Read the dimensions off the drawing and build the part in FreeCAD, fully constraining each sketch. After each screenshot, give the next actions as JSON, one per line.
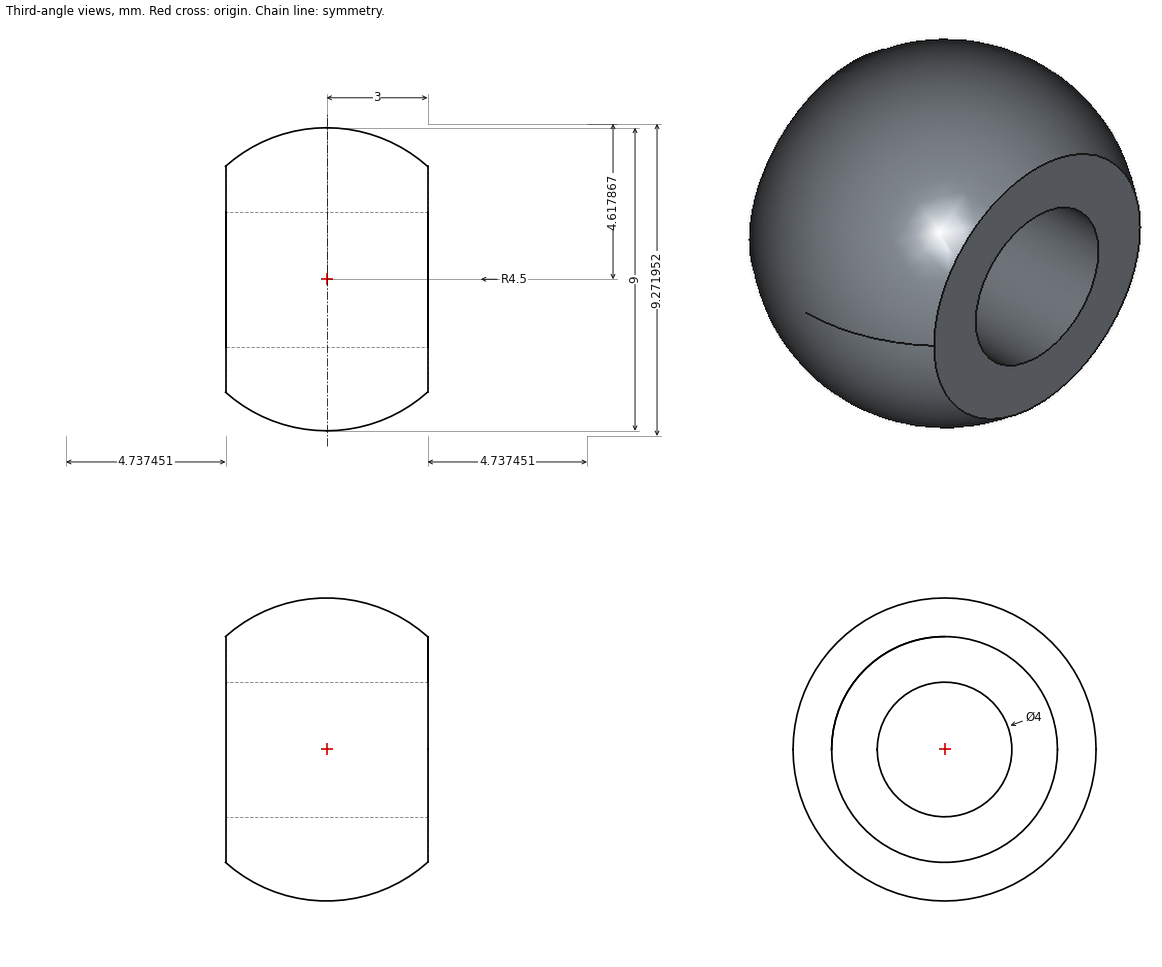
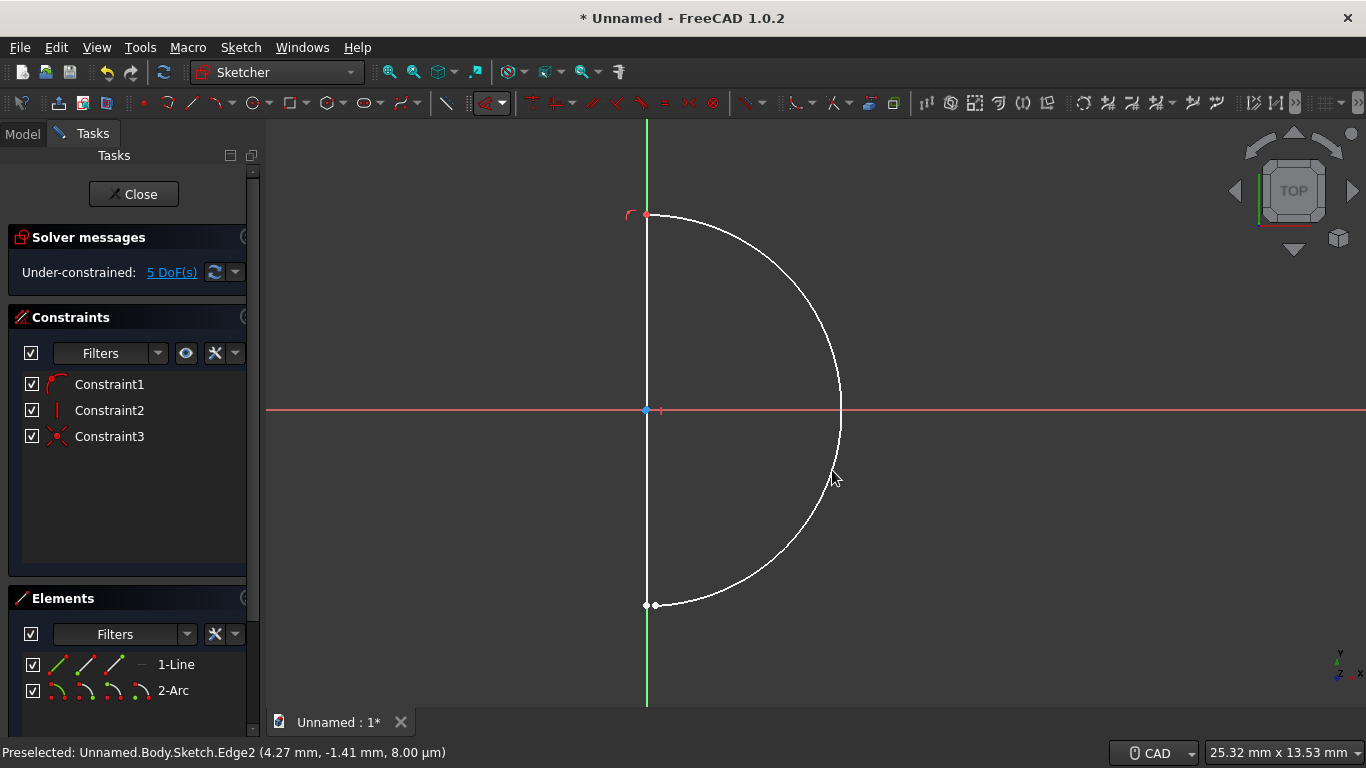
{"action": "left_click_drag", "start_coordinate": [636, 400], "coordinate": [657, 421]}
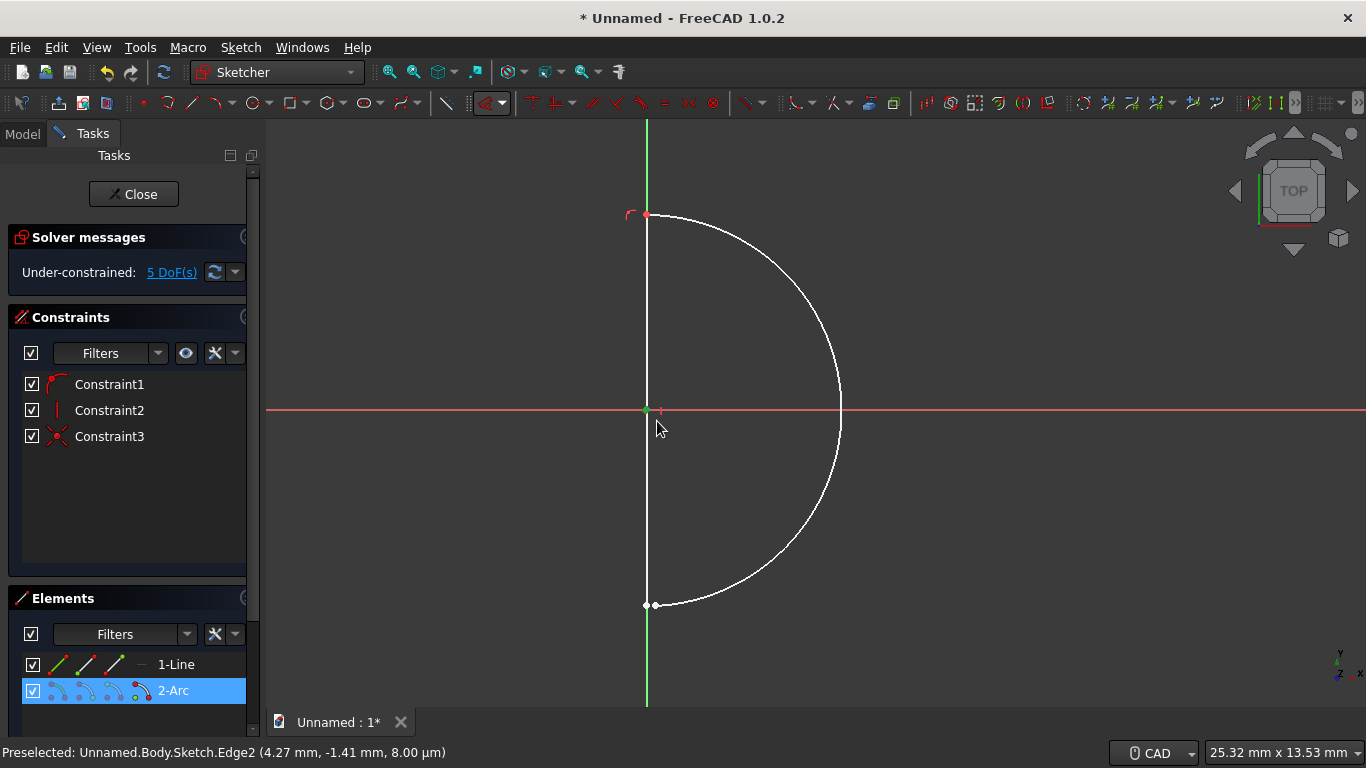
{"action": "key", "text": "c"}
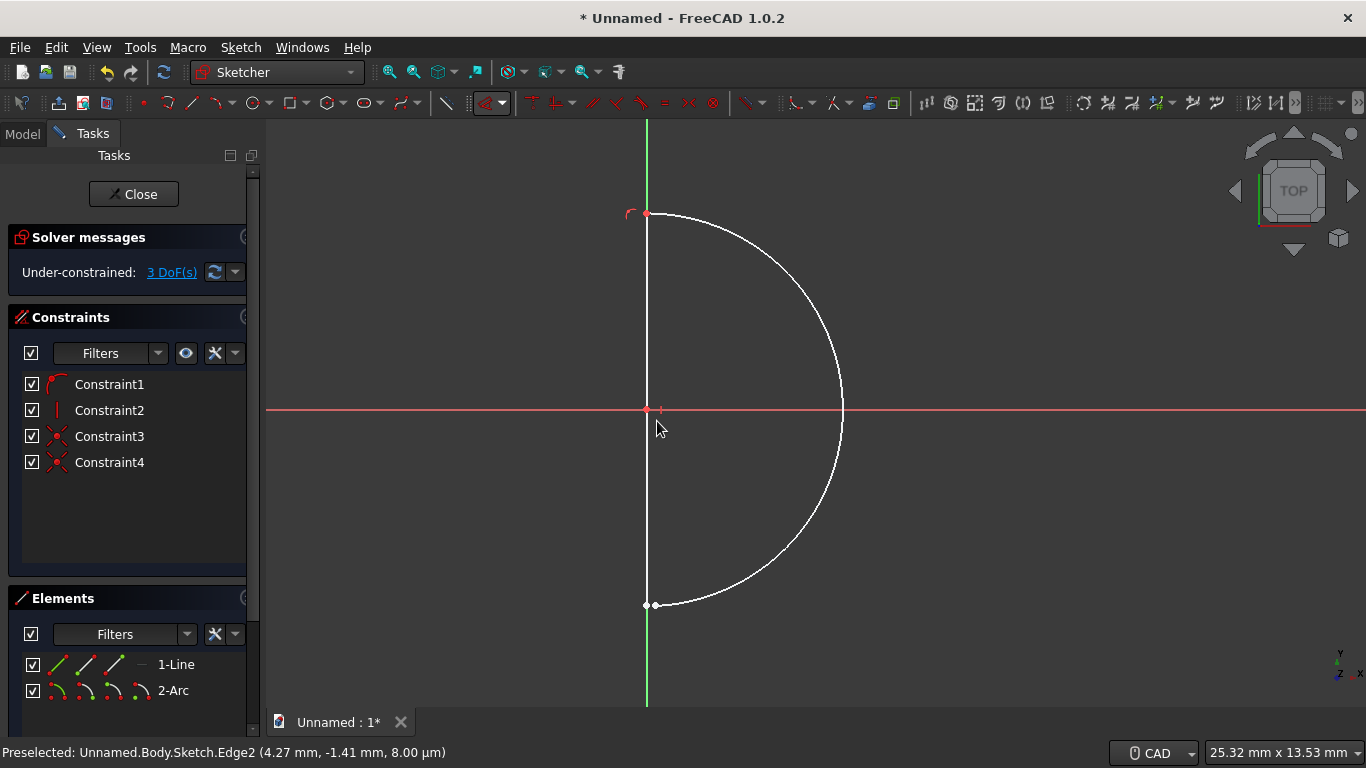
{"action": "left_click", "coordinate": [486, 104]}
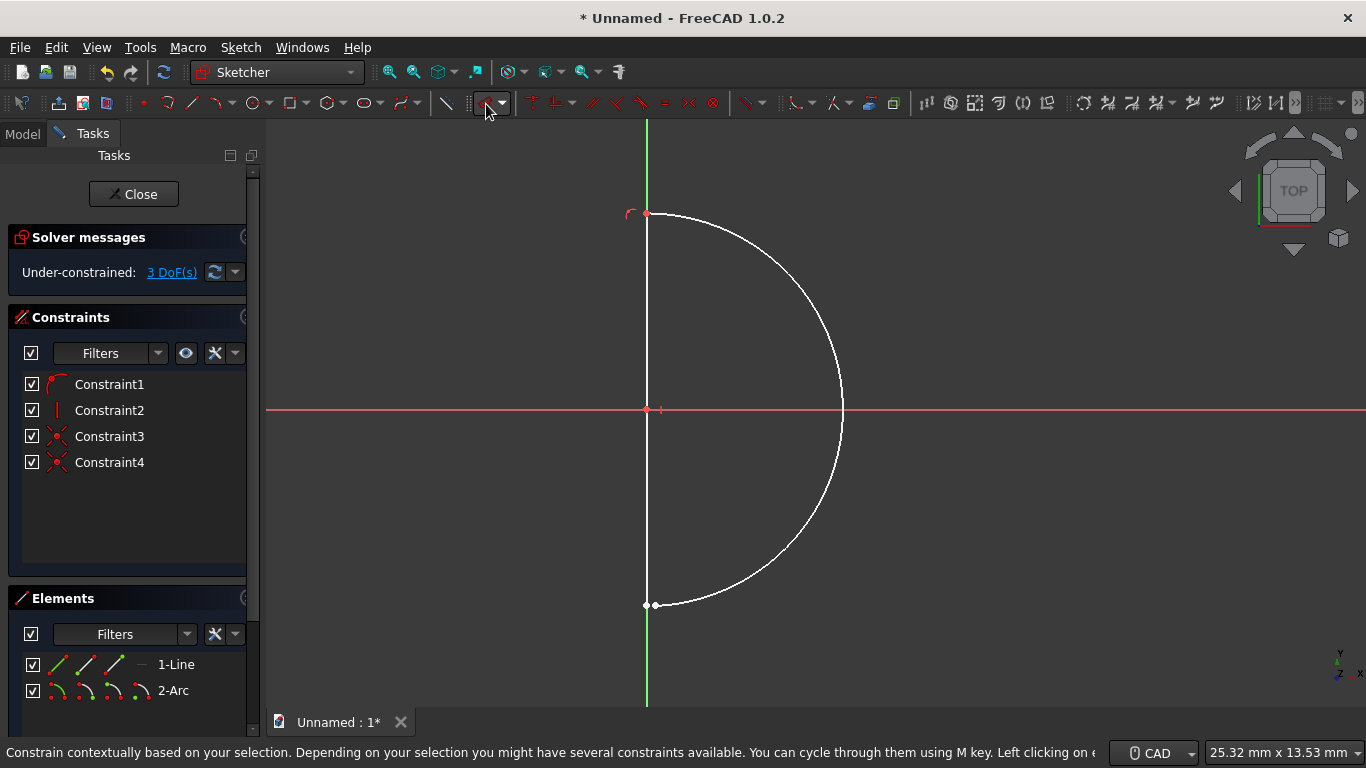
{"action": "left_click", "coordinate": [809, 520]}
{"action": "left_click", "coordinate": [835, 538]}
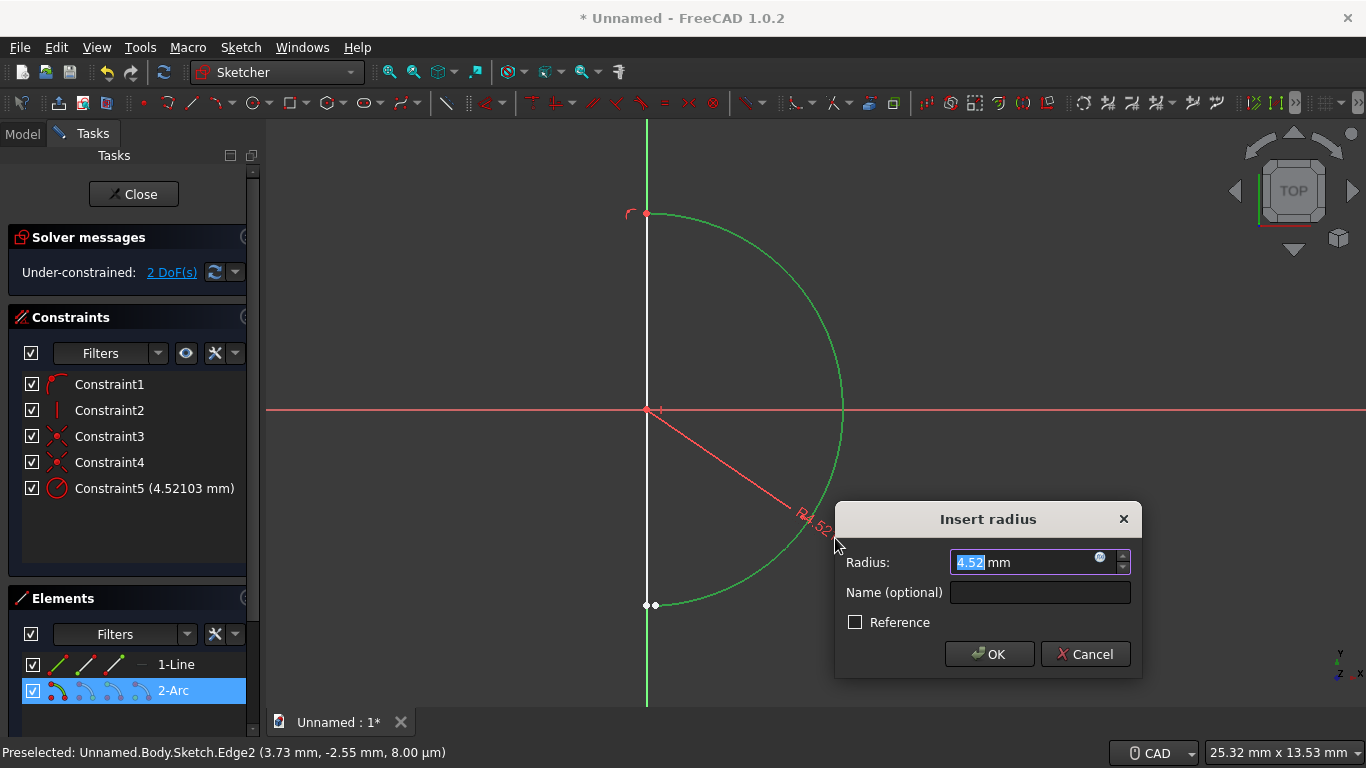
{"action": "type", "text": "4.5"}
{"action": "key", "text": "Return"}
{"action": "key", "text": "Escape"}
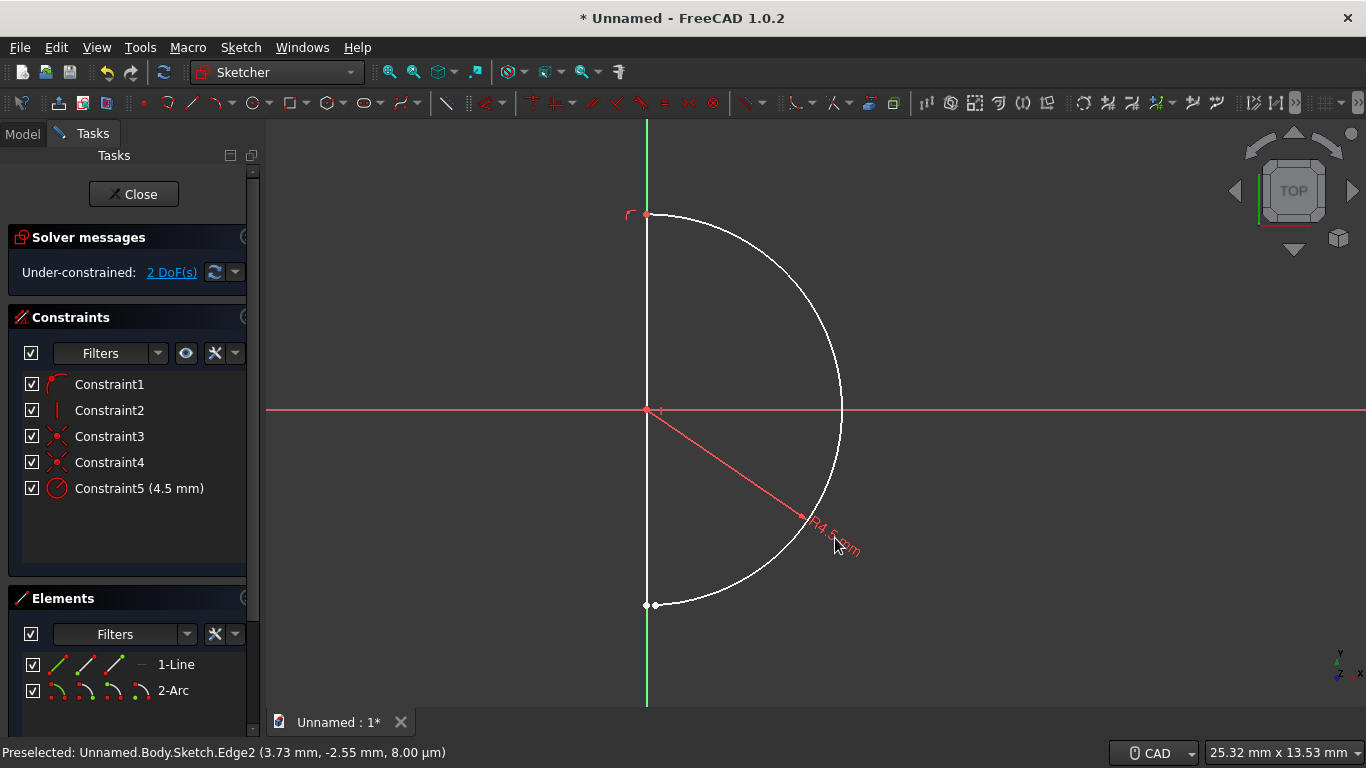
{"action": "left_click", "coordinate": [656, 605]}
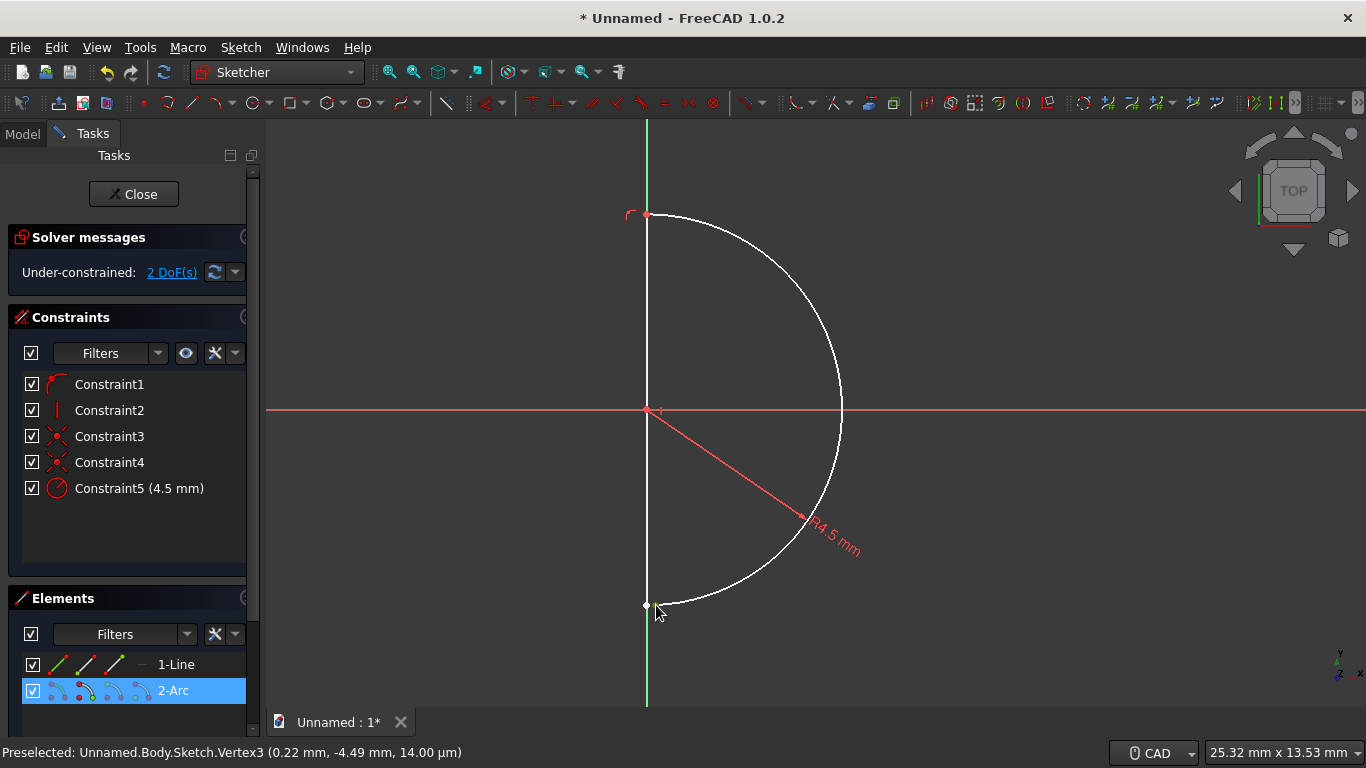
{"action": "left_click", "coordinate": [647, 641]}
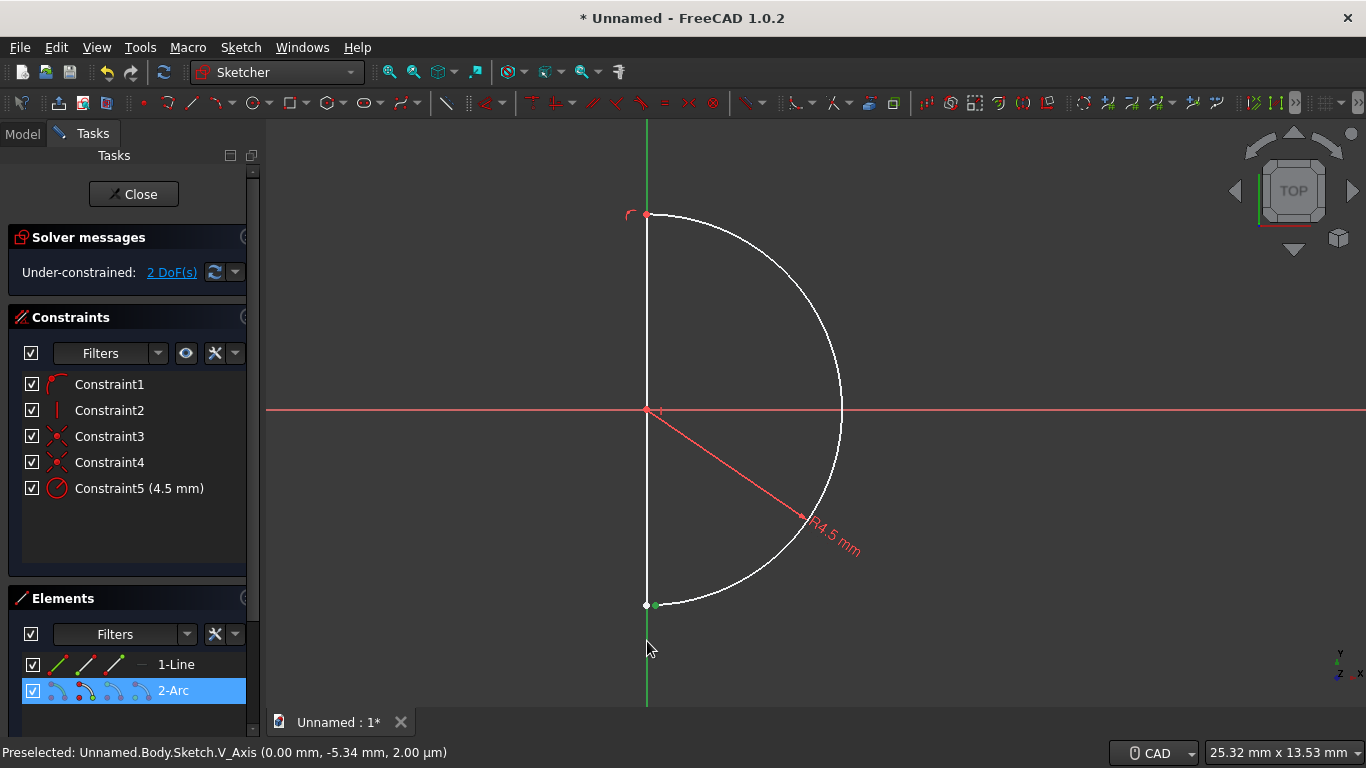
{"action": "key", "text": "c"}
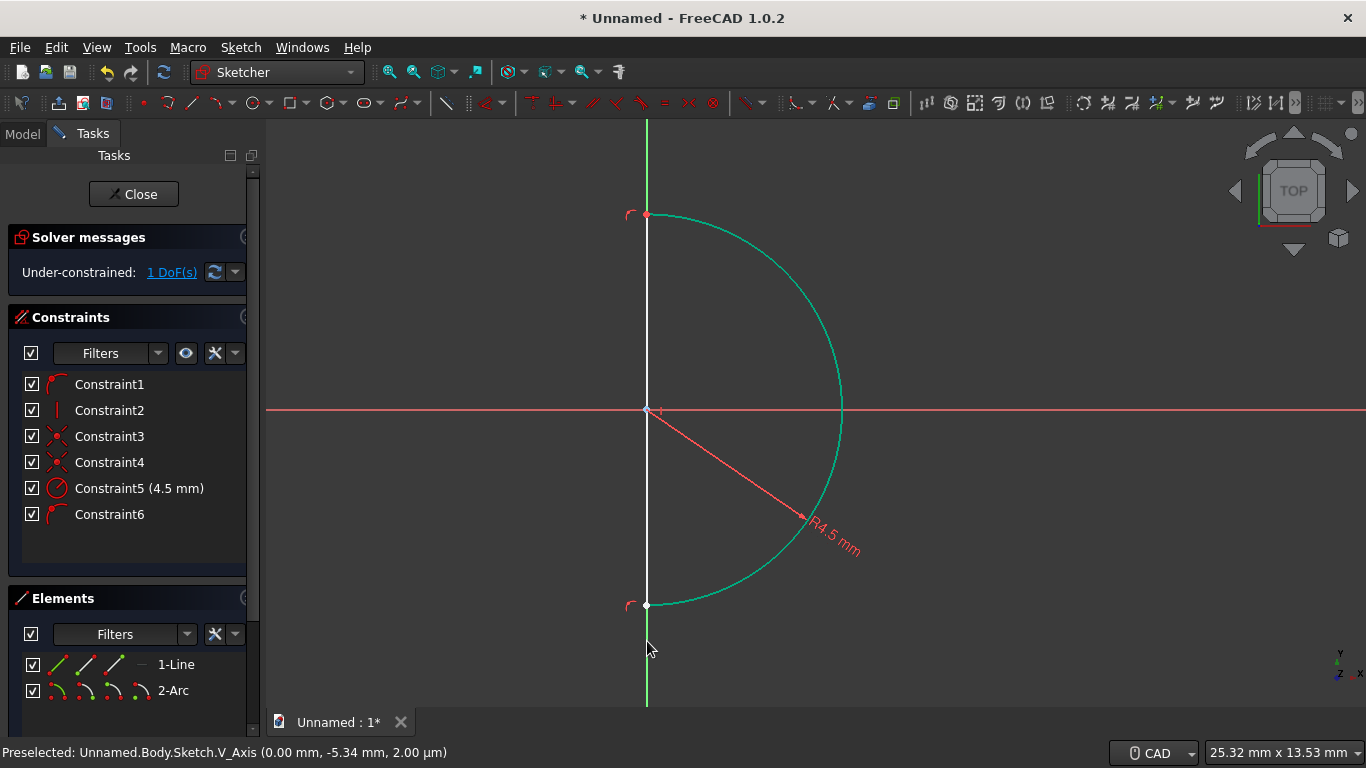
{"action": "left_click", "coordinate": [486, 104]}